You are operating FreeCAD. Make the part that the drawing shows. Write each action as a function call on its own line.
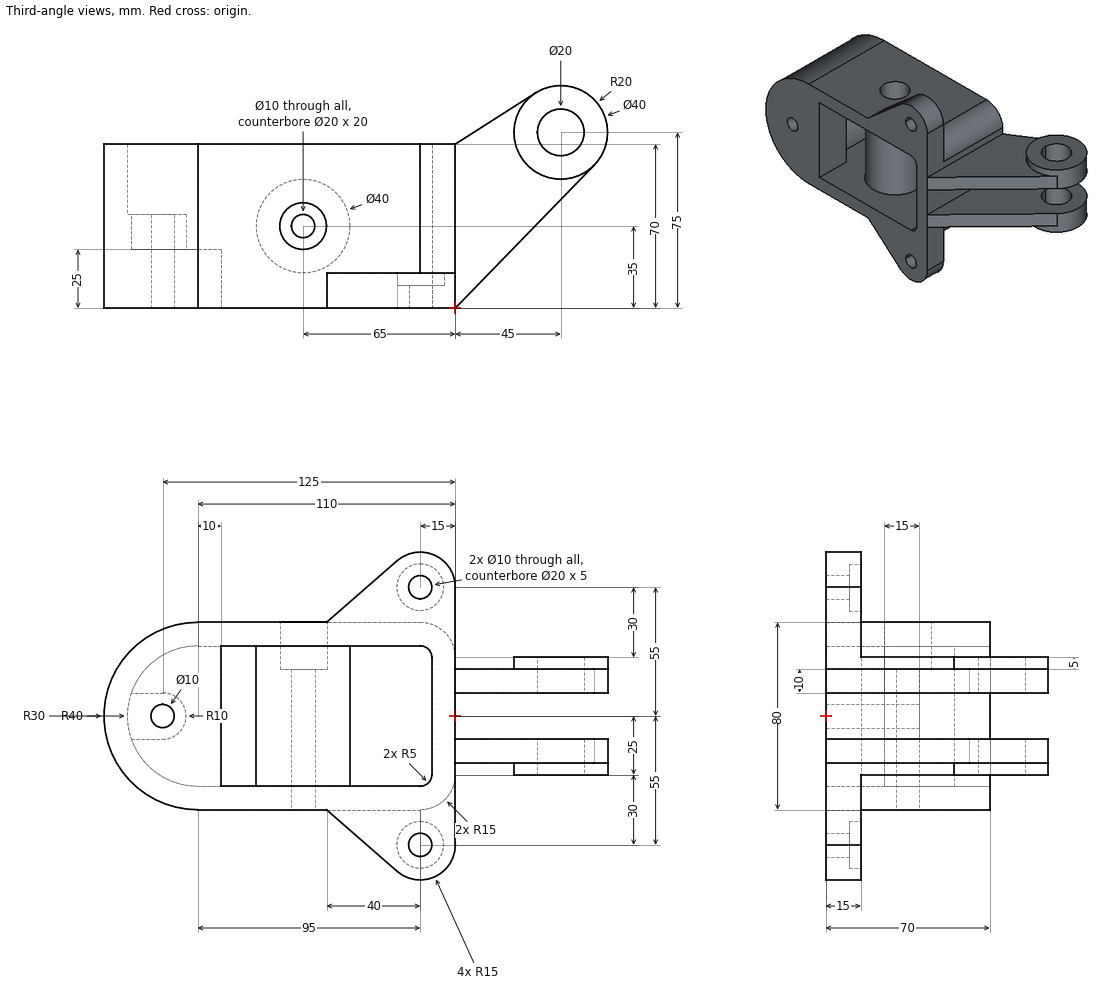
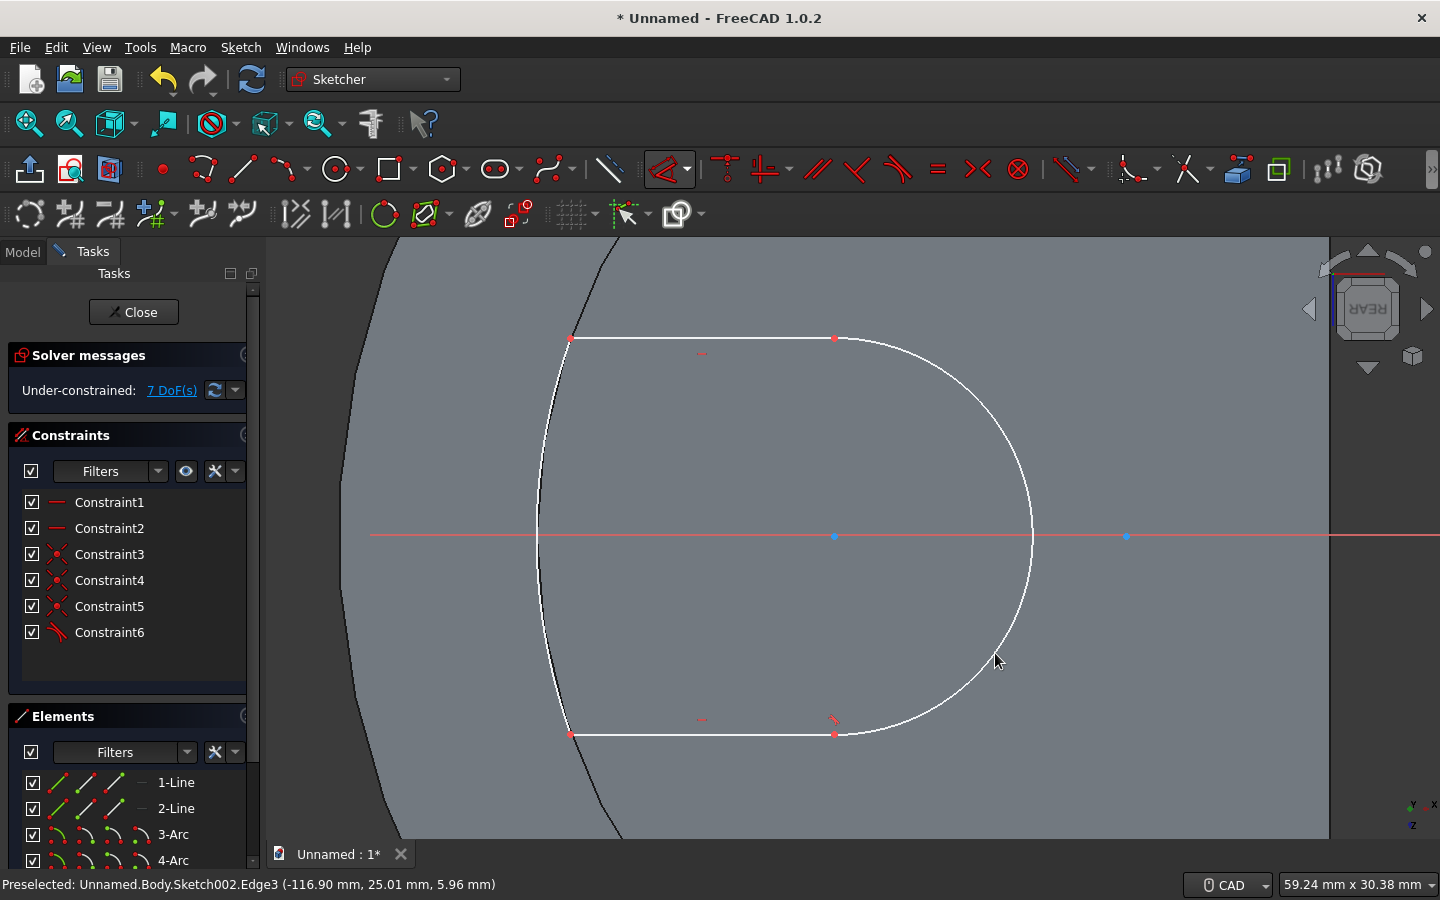
click(755, 338)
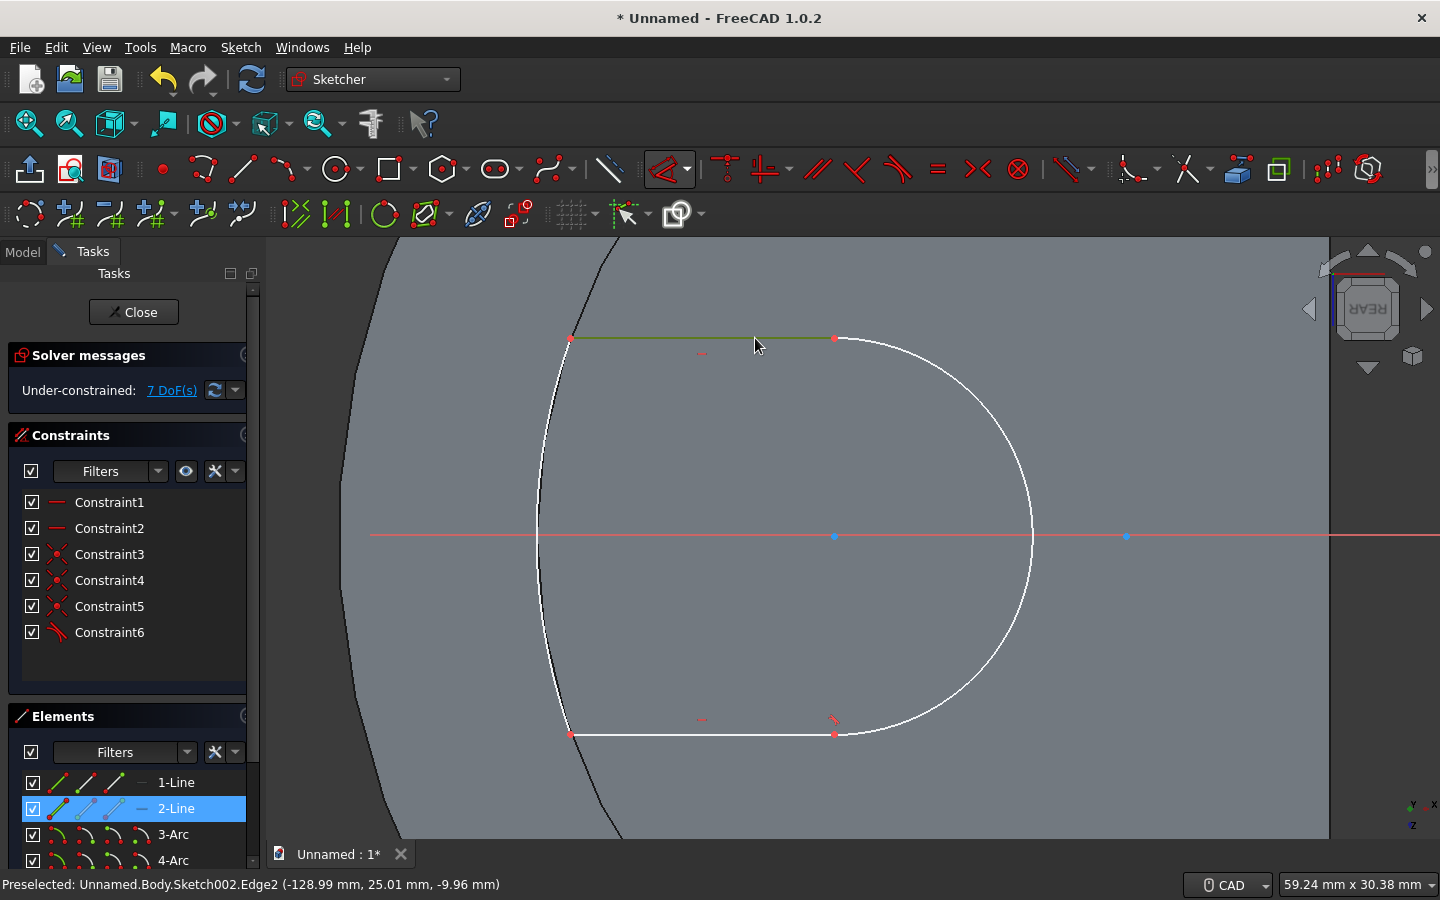
click(995, 653)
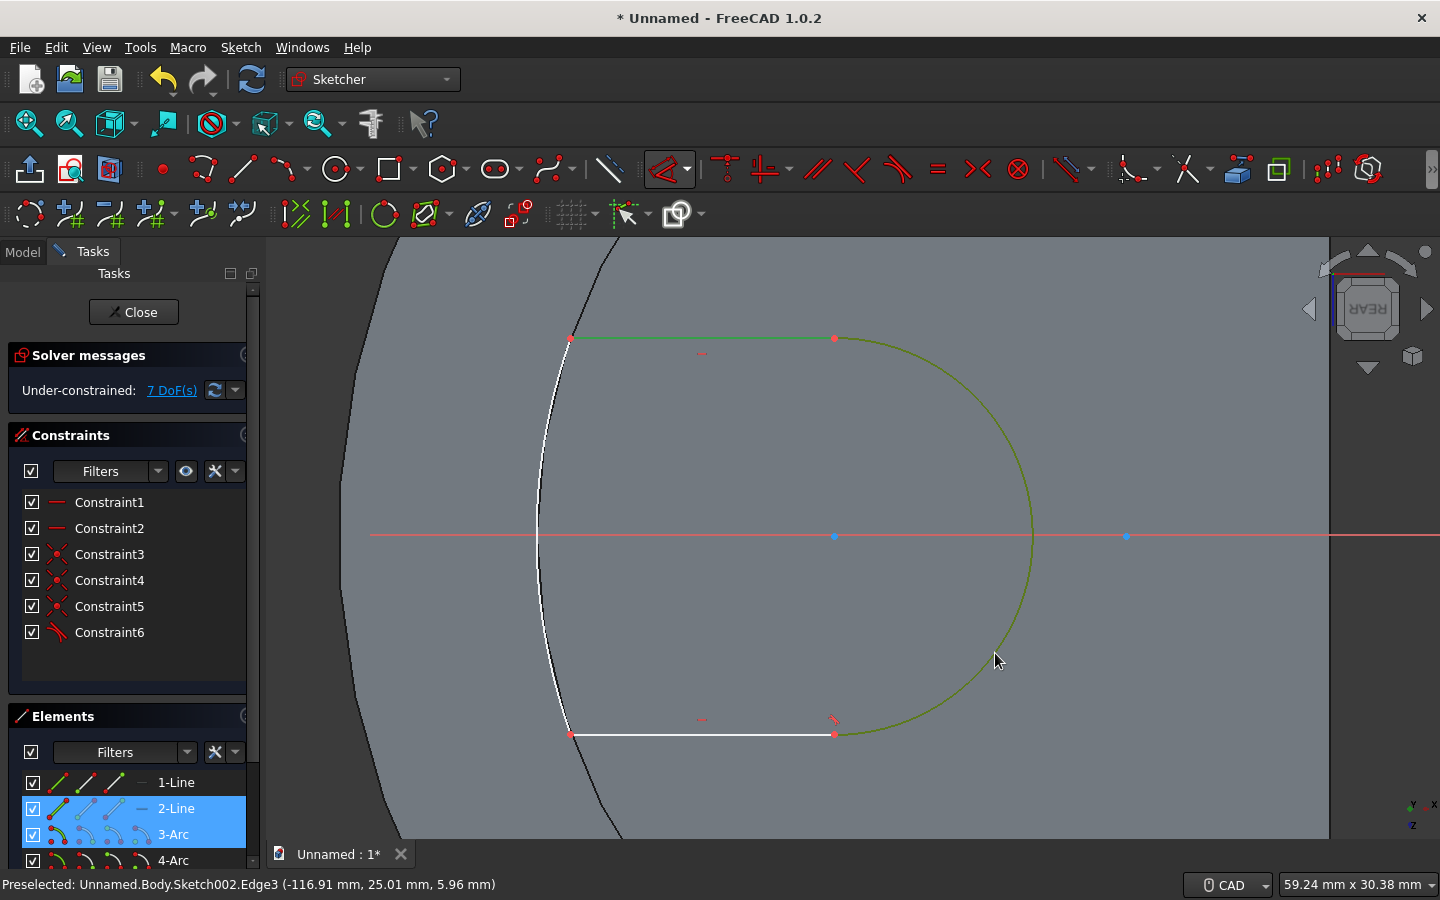
key(t)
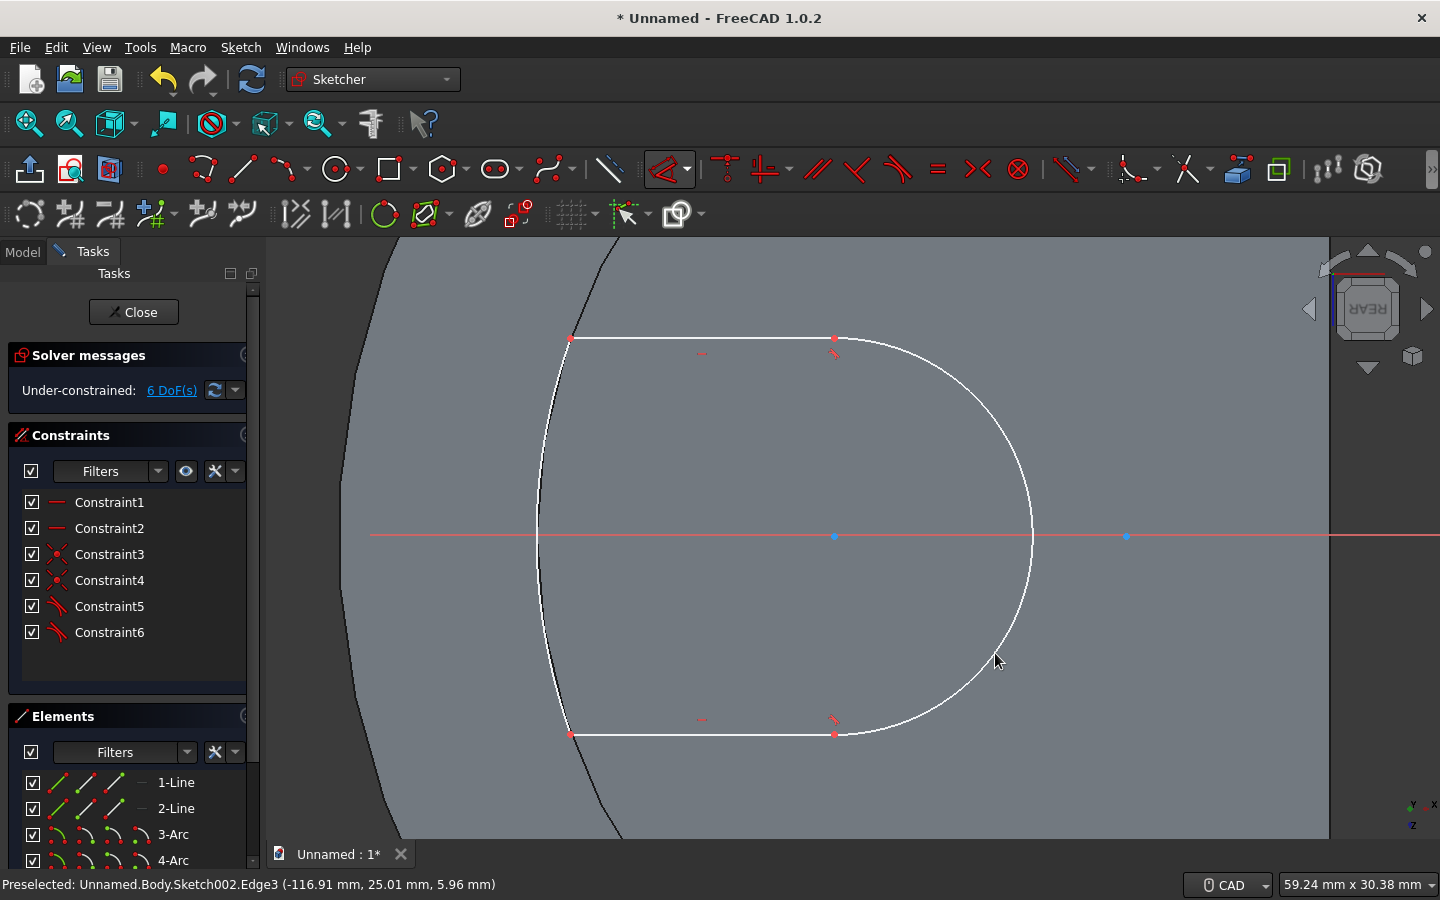
click(834, 537)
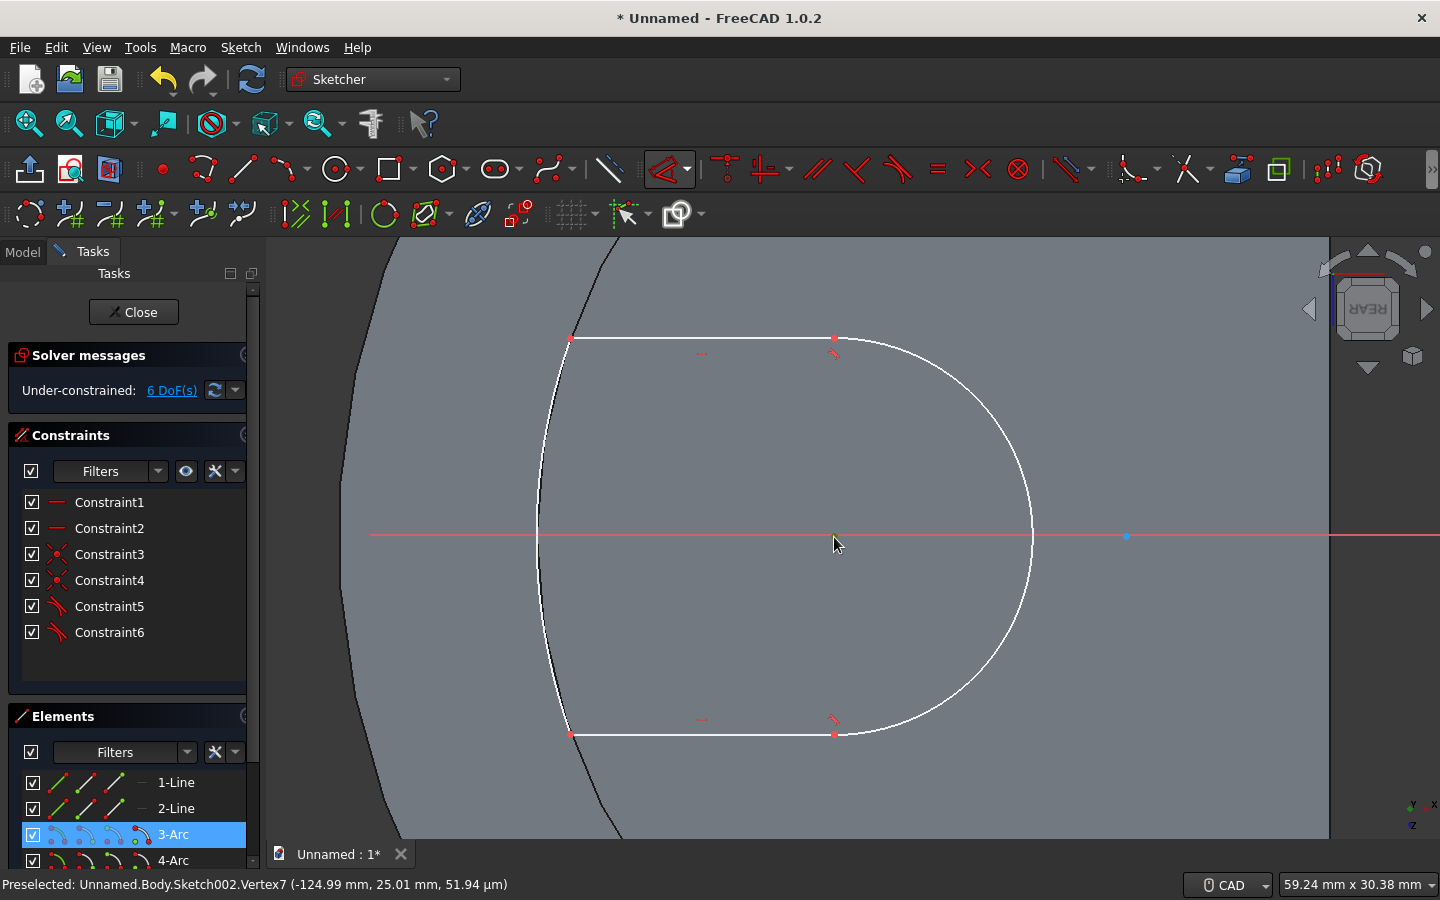
click(434, 535)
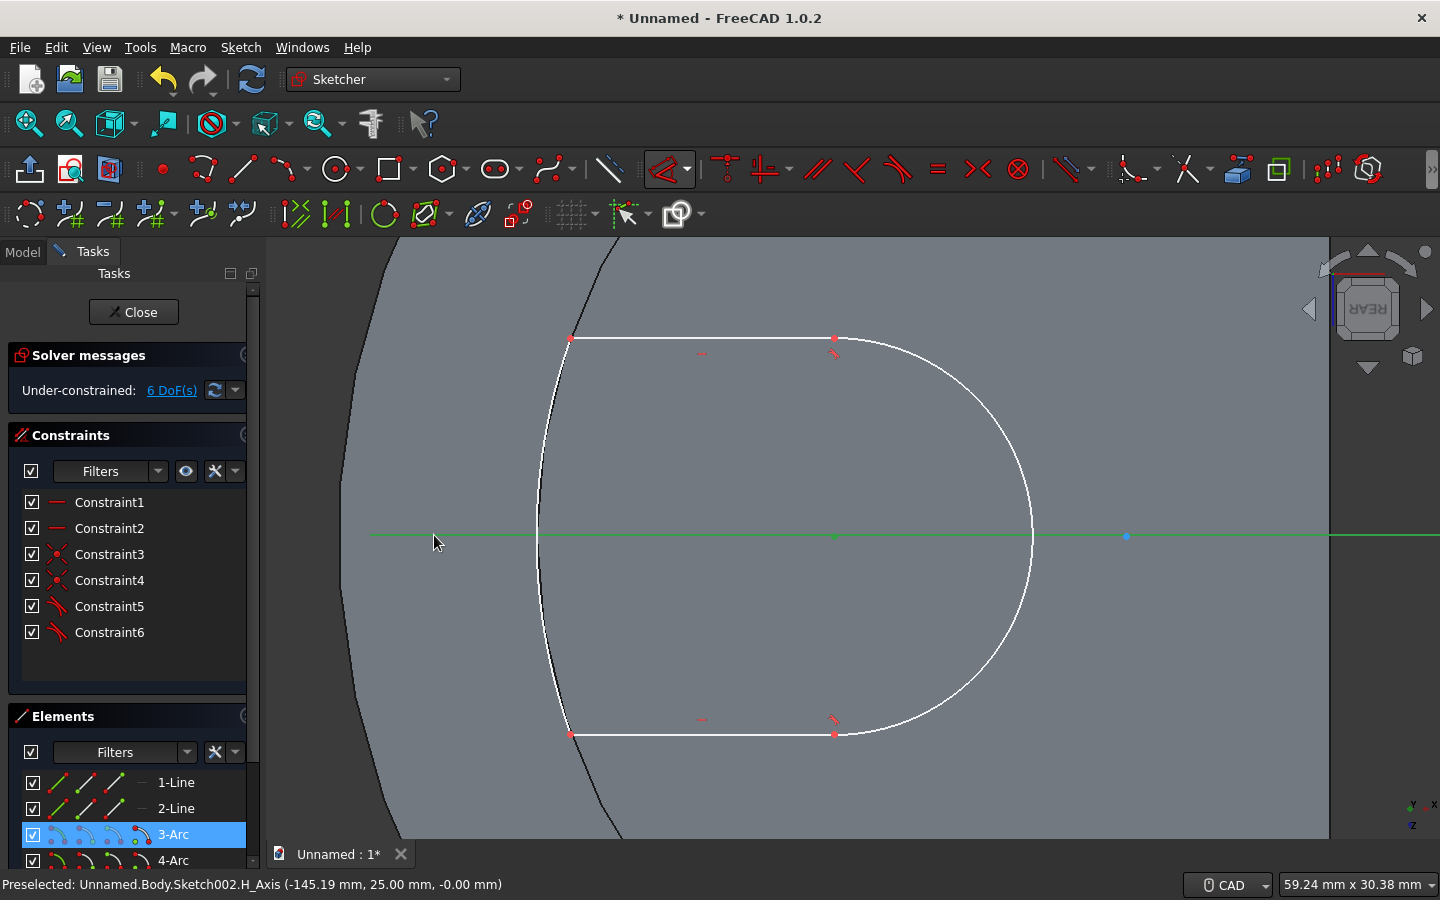
click(726, 170)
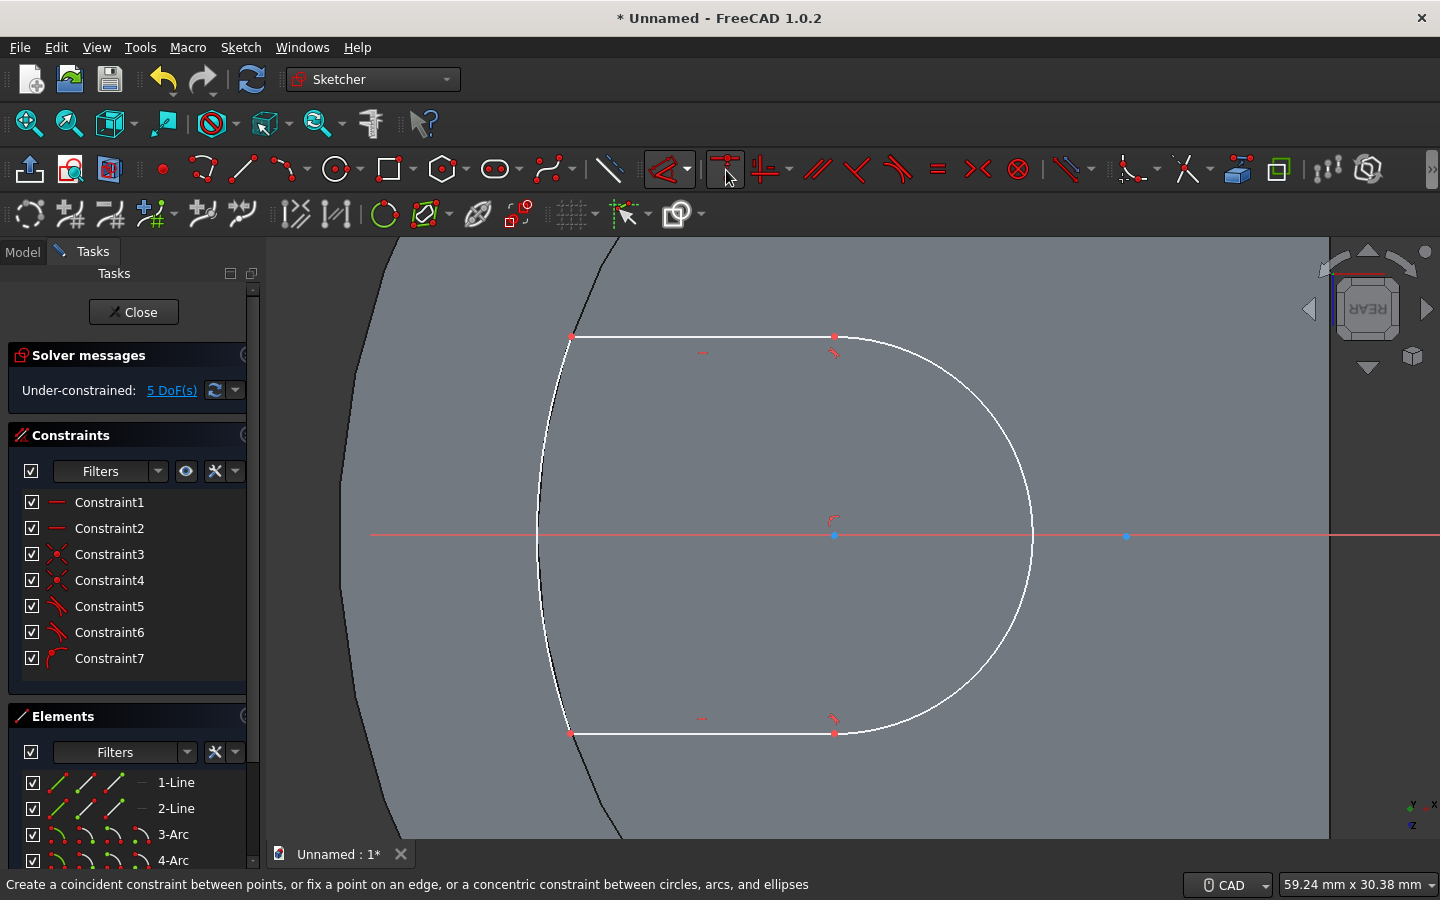
click(1127, 537)